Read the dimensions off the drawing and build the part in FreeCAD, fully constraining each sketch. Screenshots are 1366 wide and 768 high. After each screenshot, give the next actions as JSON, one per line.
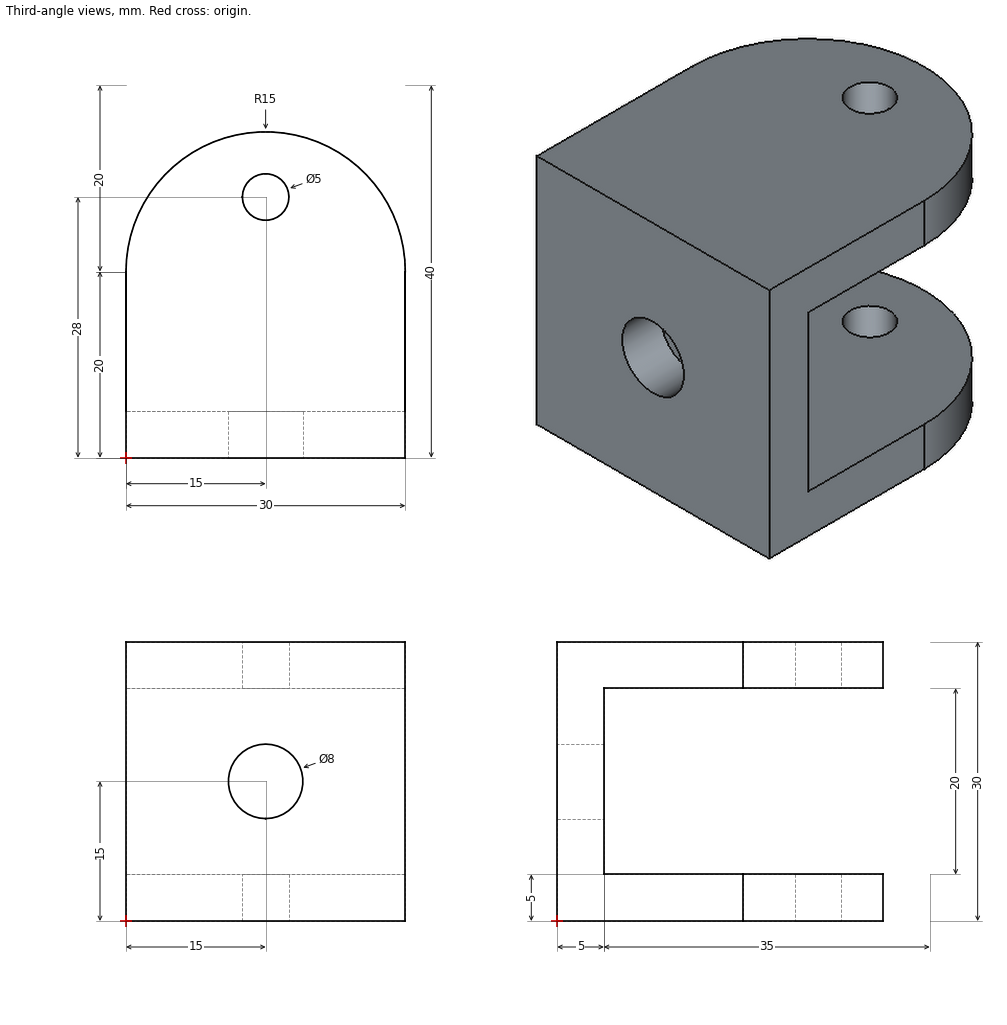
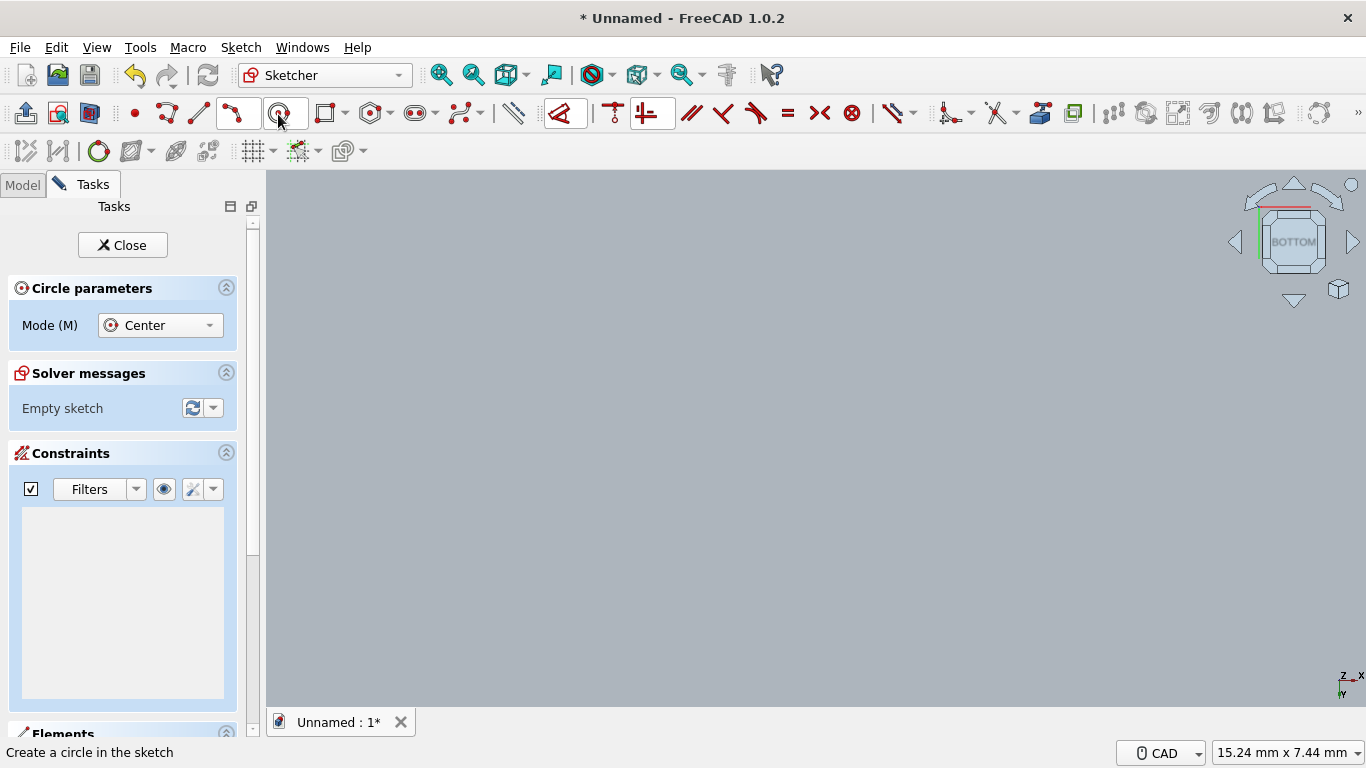
{"action": "left_click", "coordinate": [742, 436]}
{"action": "mouse_move", "coordinate": [870, 308]}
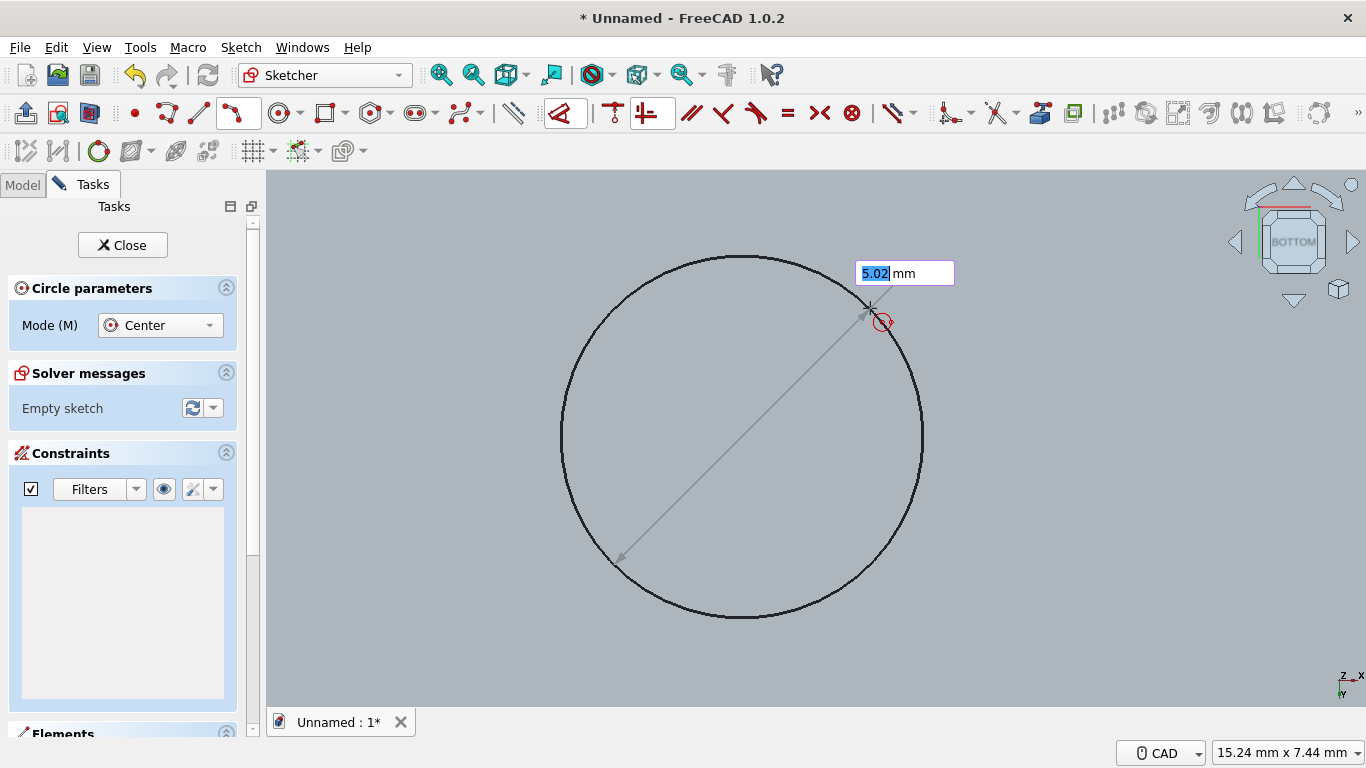
{"action": "type", "text": "5"}
{"action": "key", "text": "Return"}
{"action": "key", "text": "Escape"}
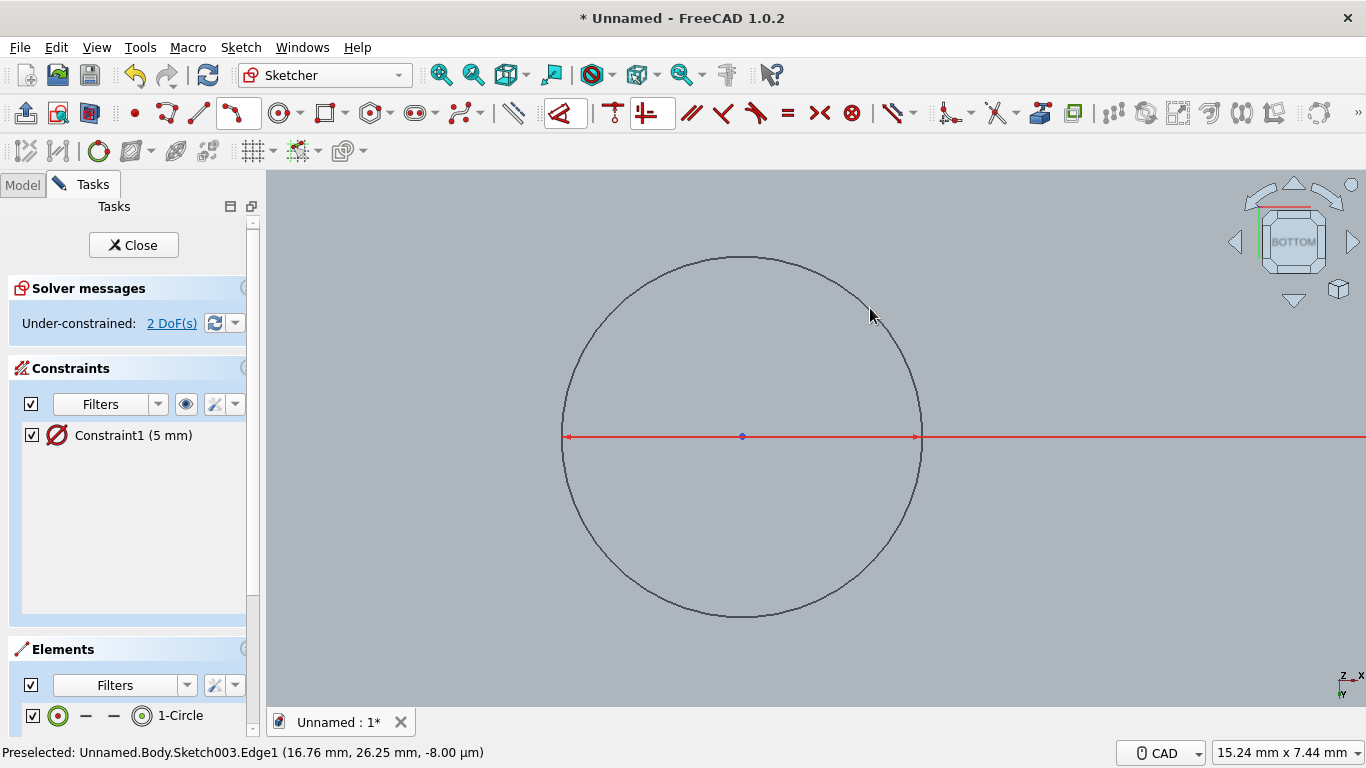
{"action": "left_click", "coordinate": [742, 437]}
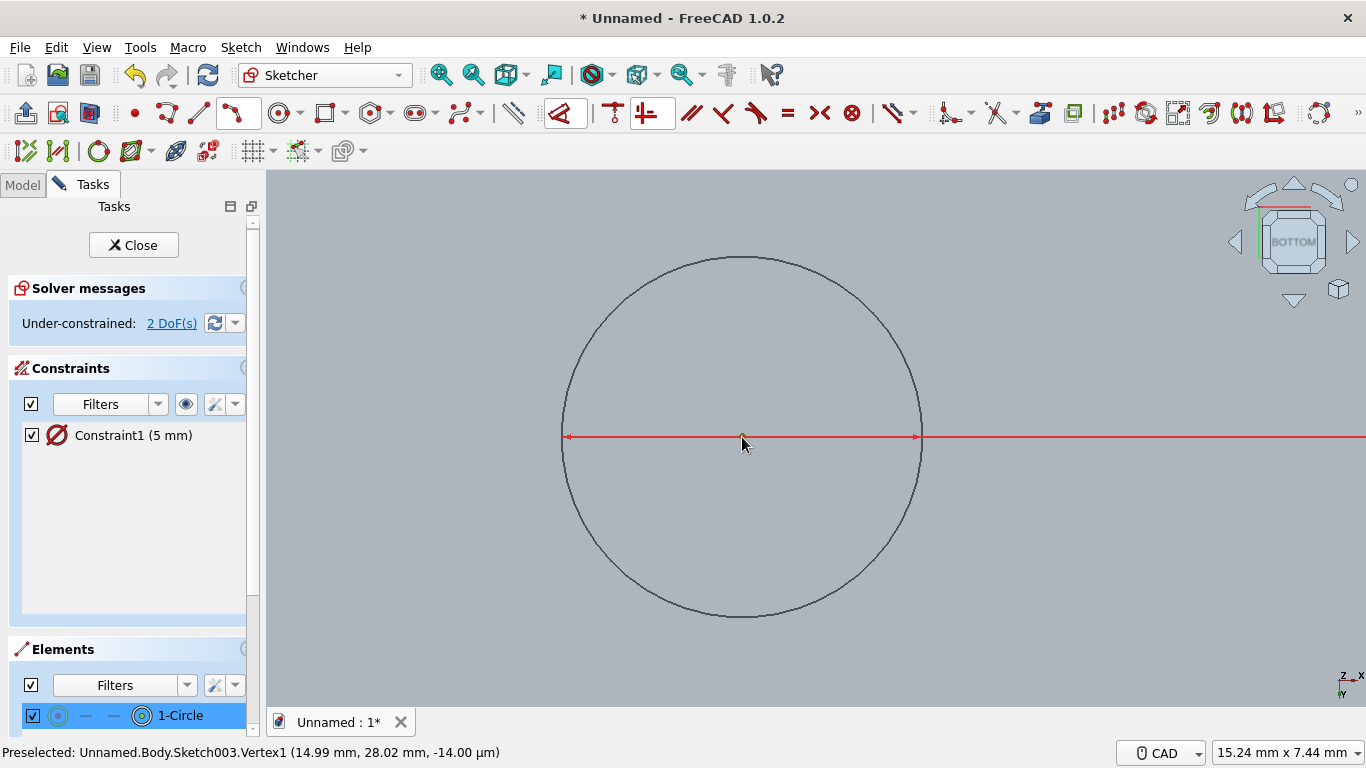
{"action": "key", "text": "l"}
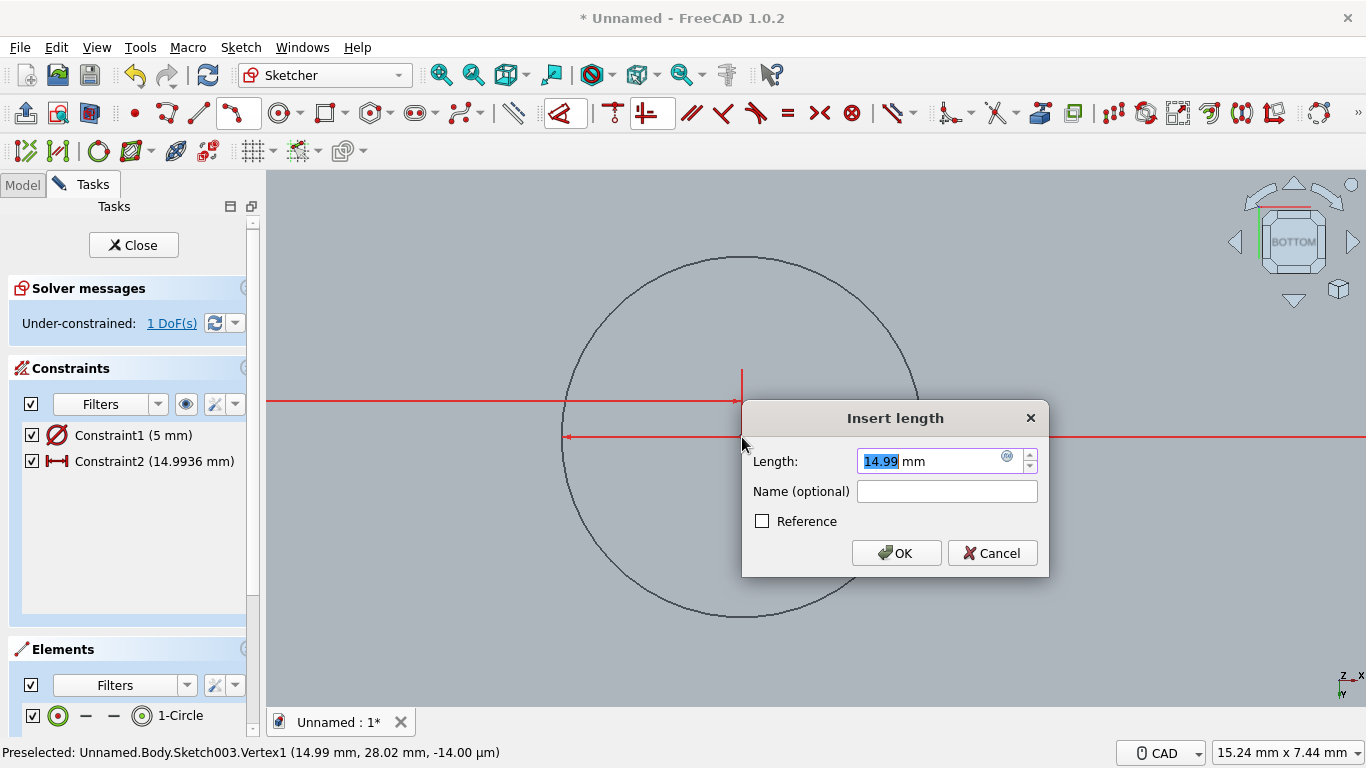
{"action": "type", "text": "15"}
{"action": "key", "text": "Return"}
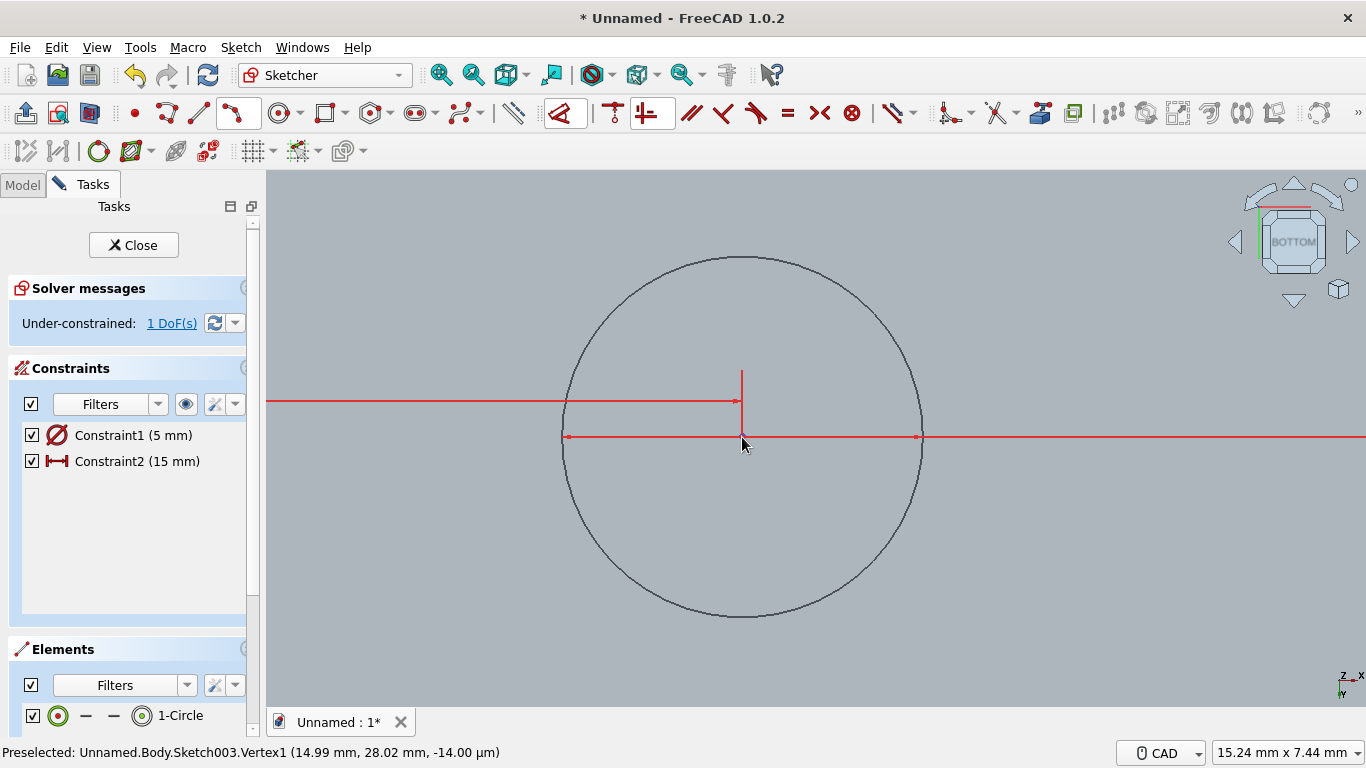
{"action": "left_click", "coordinate": [742, 437]}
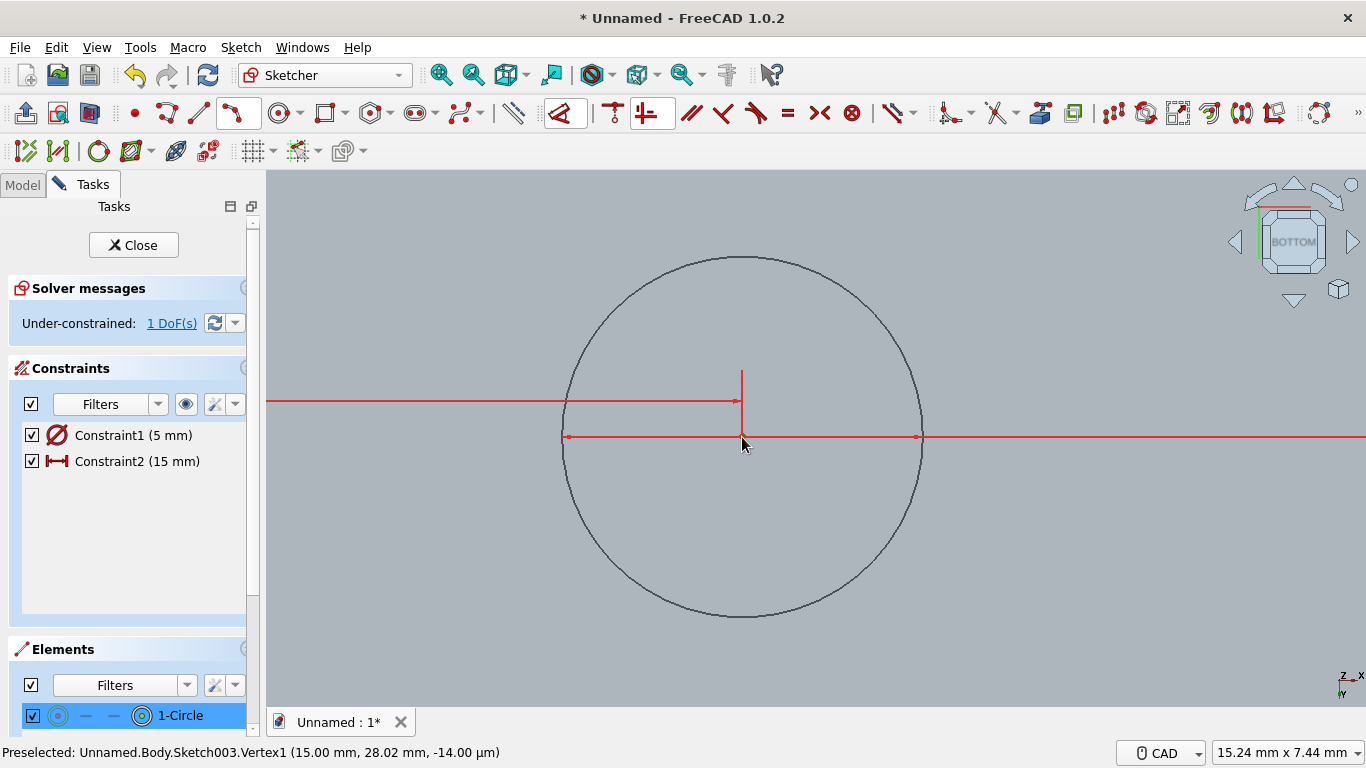
{"action": "left_click", "coordinate": [582, 114]}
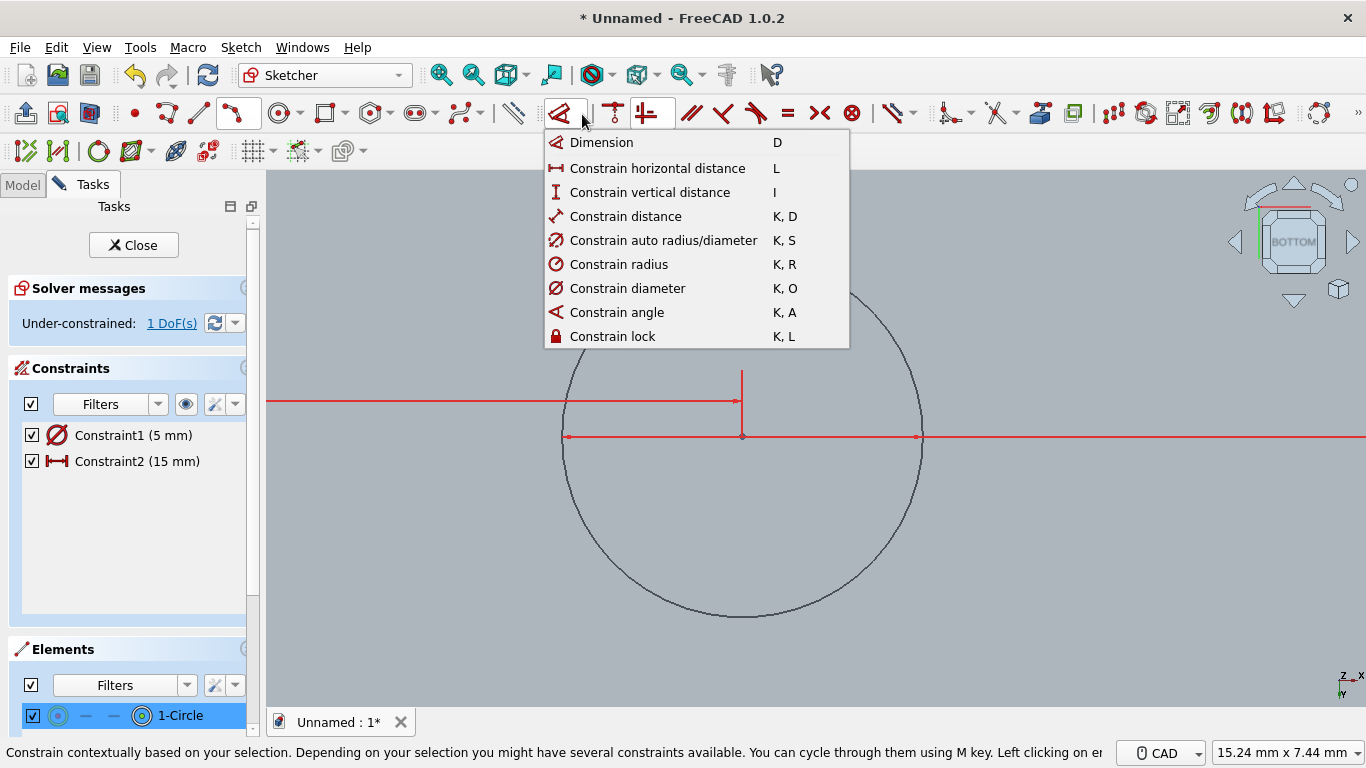
{"action": "left_click", "coordinate": [697, 192]}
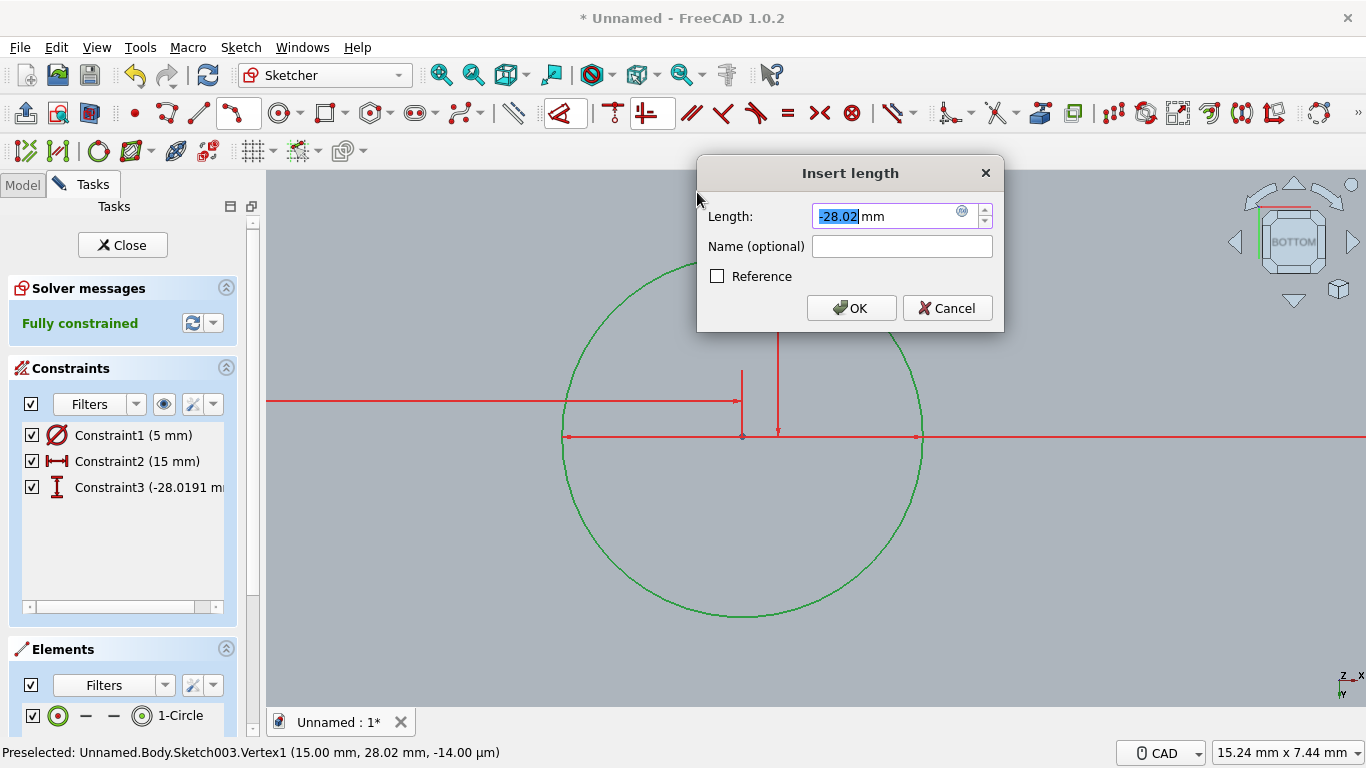
{"action": "type", "text": "-28"}
{"action": "key", "text": "Return"}